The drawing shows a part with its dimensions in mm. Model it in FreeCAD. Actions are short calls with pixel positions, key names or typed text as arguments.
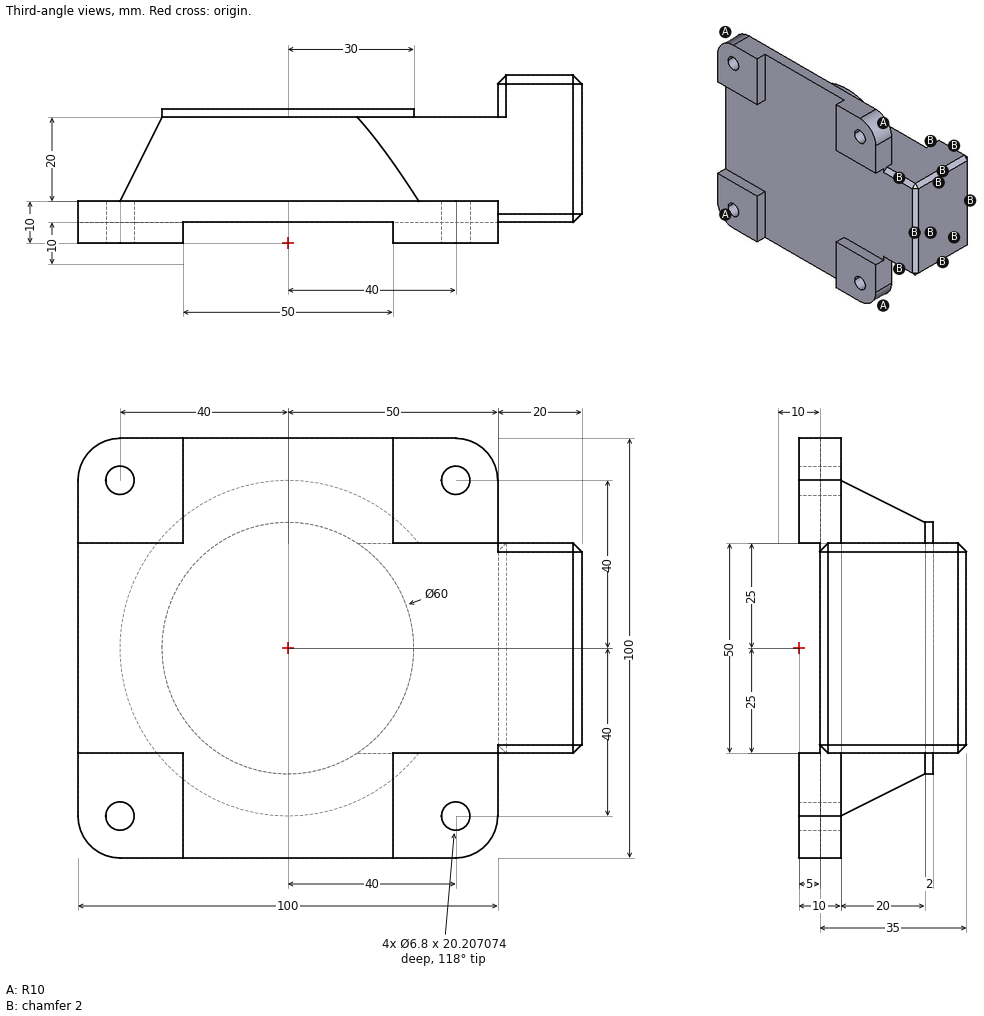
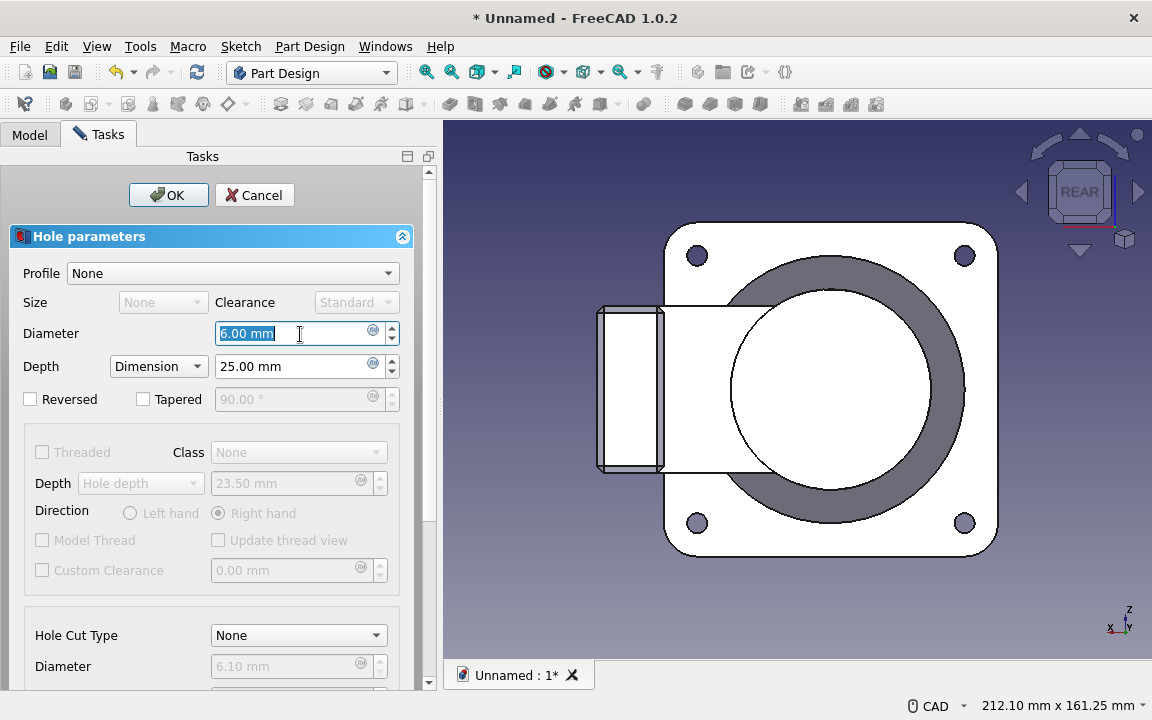
text(6.8)
key(Tab)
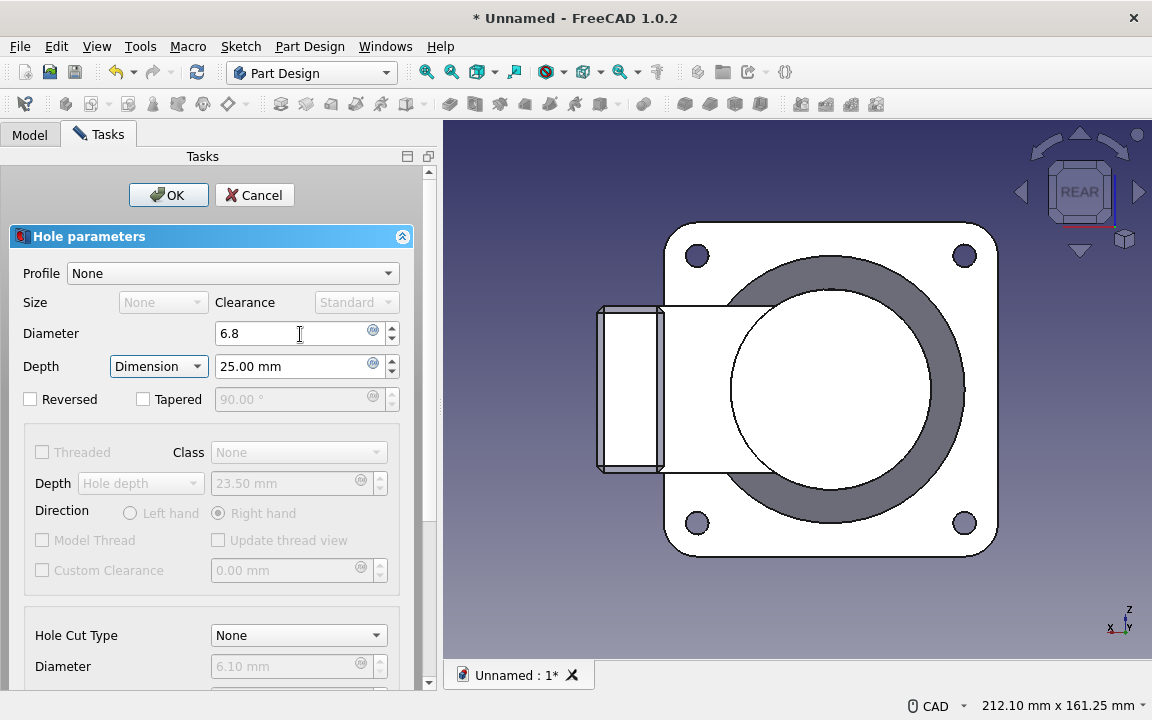
triple_click(300, 366)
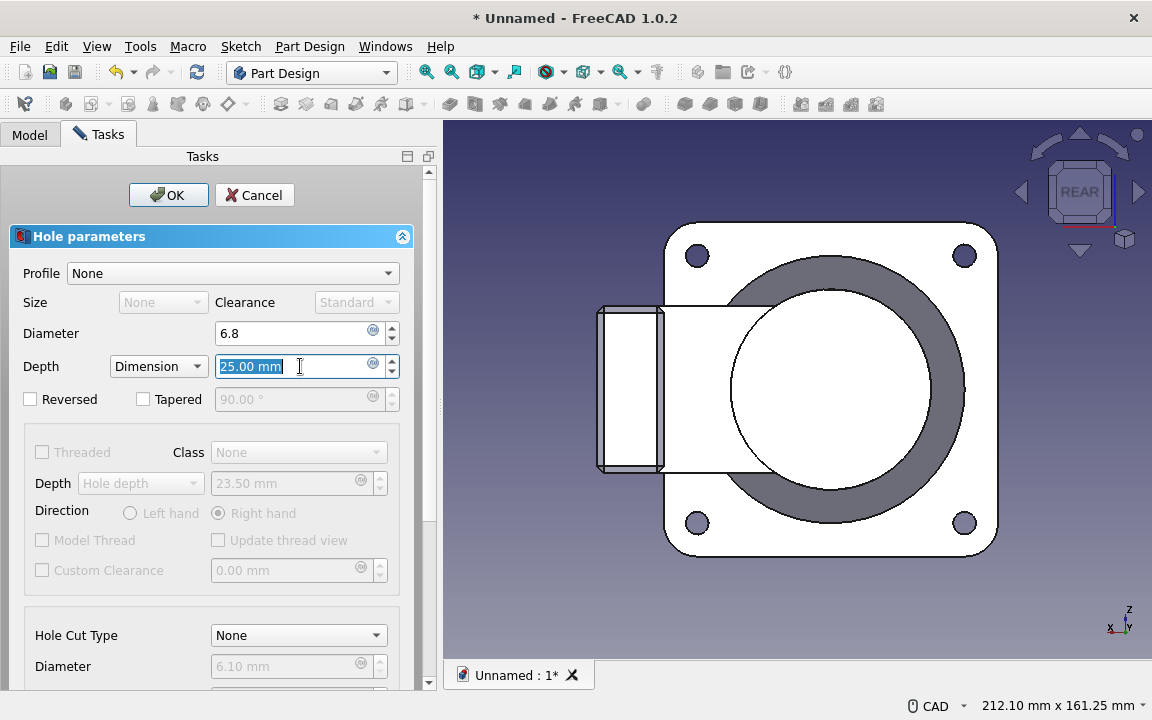
text(20.207074)
key(Tab)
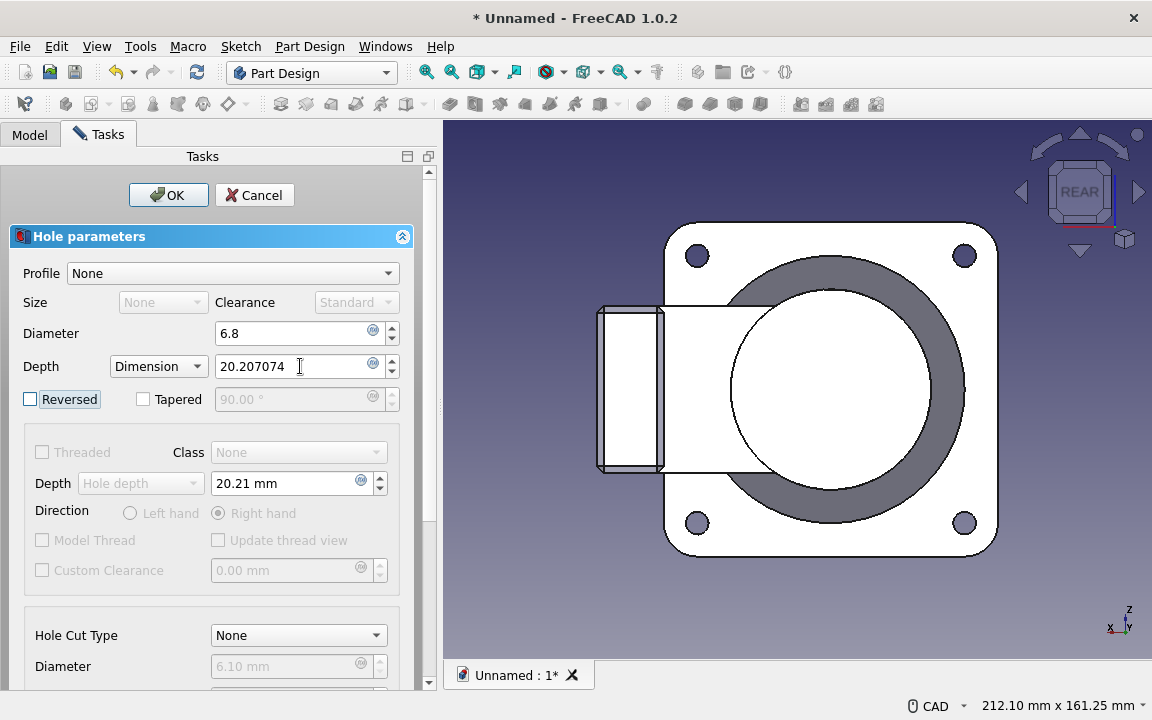
click(169, 195)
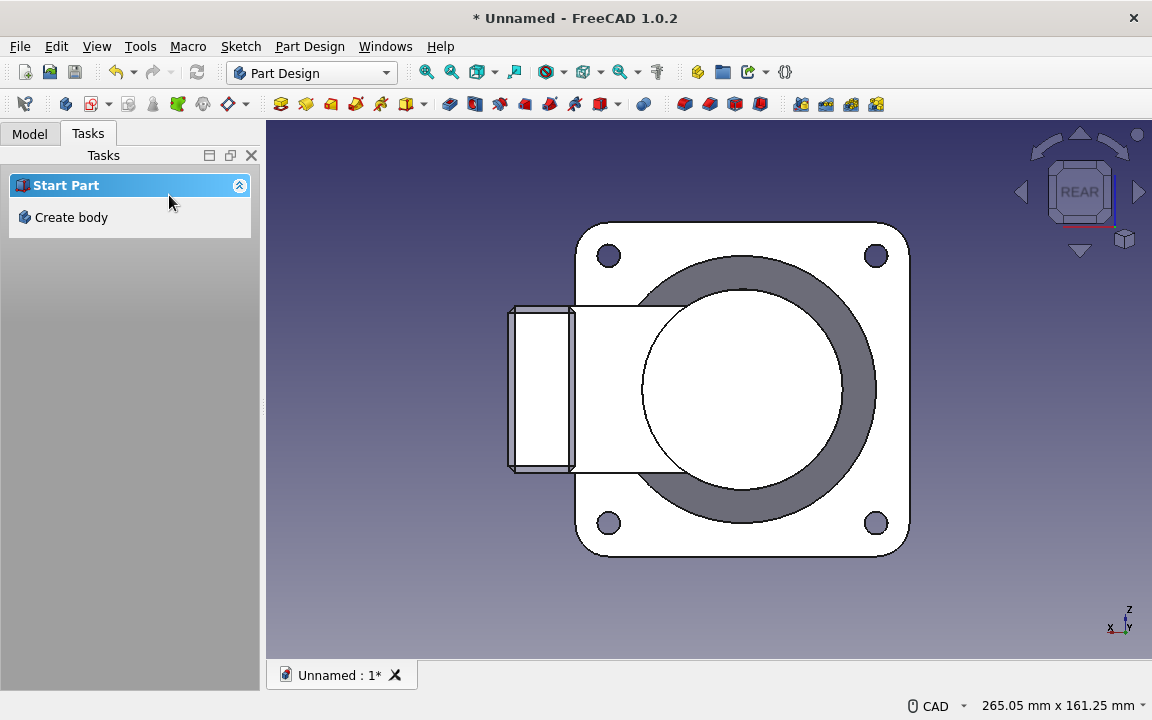
key(0)